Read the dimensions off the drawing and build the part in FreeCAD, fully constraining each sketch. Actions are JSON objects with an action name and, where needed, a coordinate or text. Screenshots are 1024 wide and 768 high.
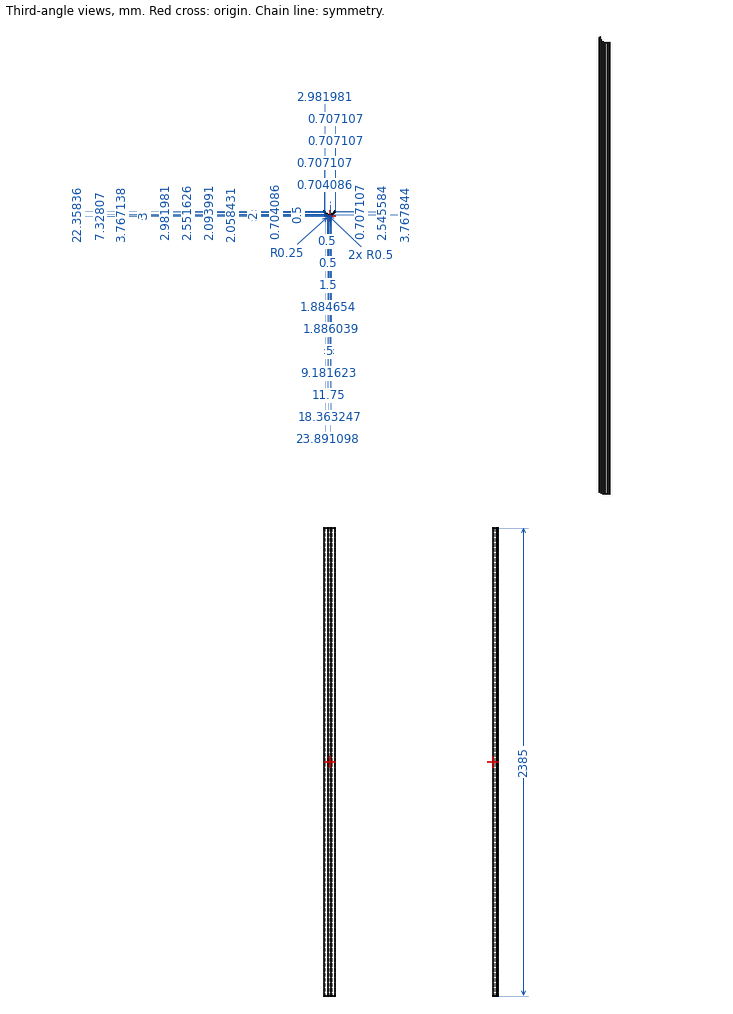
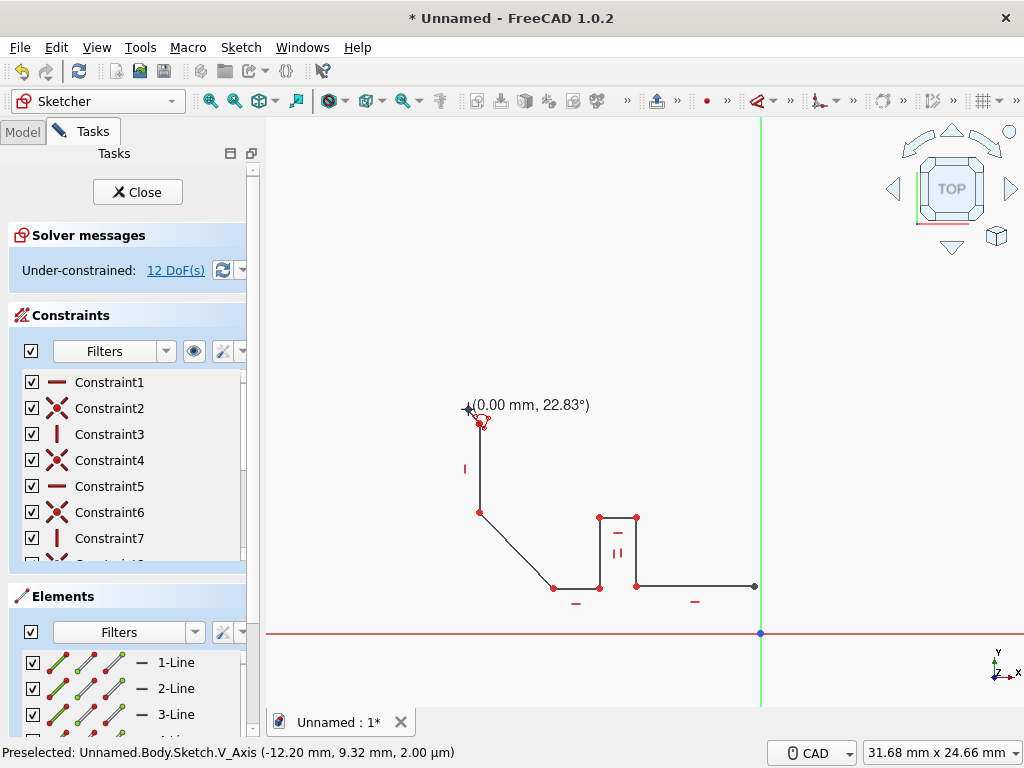
{"action": "scroll", "coordinate": [456, 409], "scroll_direction": "up", "scroll_amount": 2}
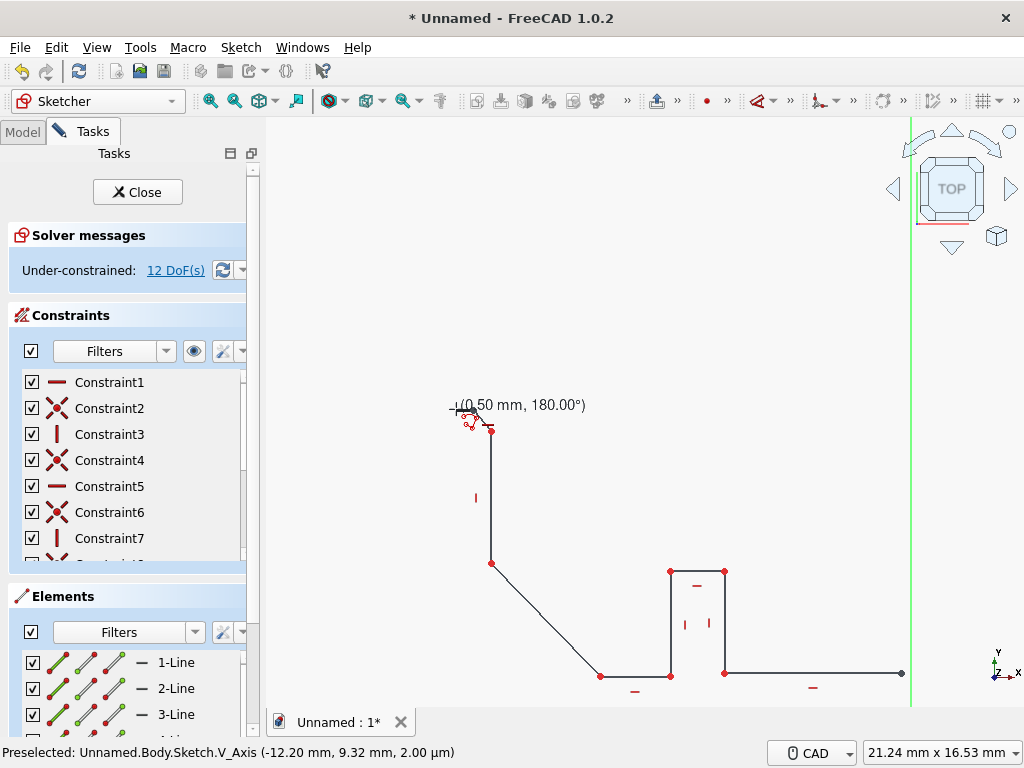
{"action": "left_click", "coordinate": [455, 409]}
{"action": "left_click", "coordinate": [455, 483]}
{"action": "right_click", "coordinate": [455, 483]}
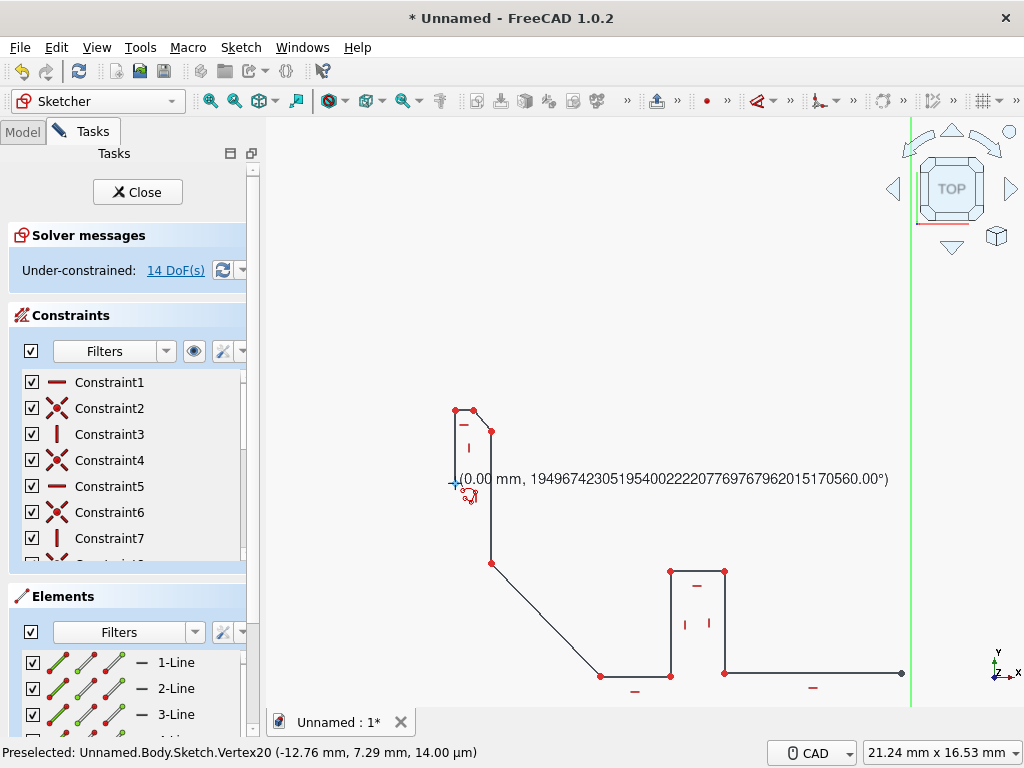
{"action": "left_click", "coordinate": [425, 495]}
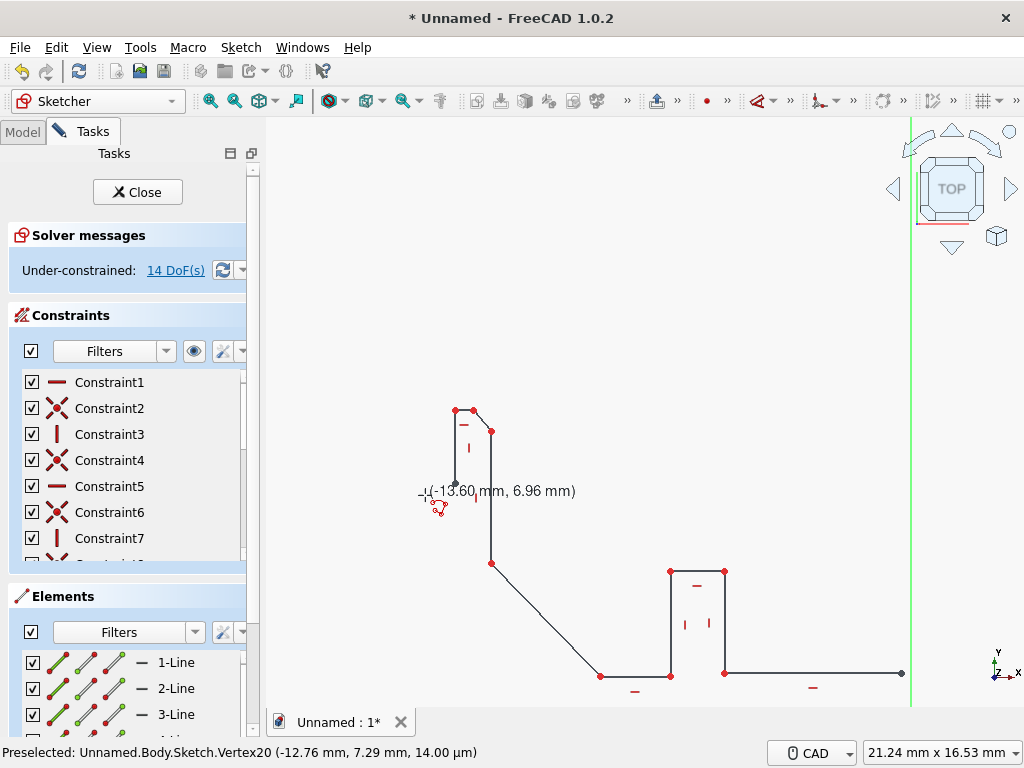
{"action": "scroll", "coordinate": [492, 429], "scroll_direction": "down", "scroll_amount": 8}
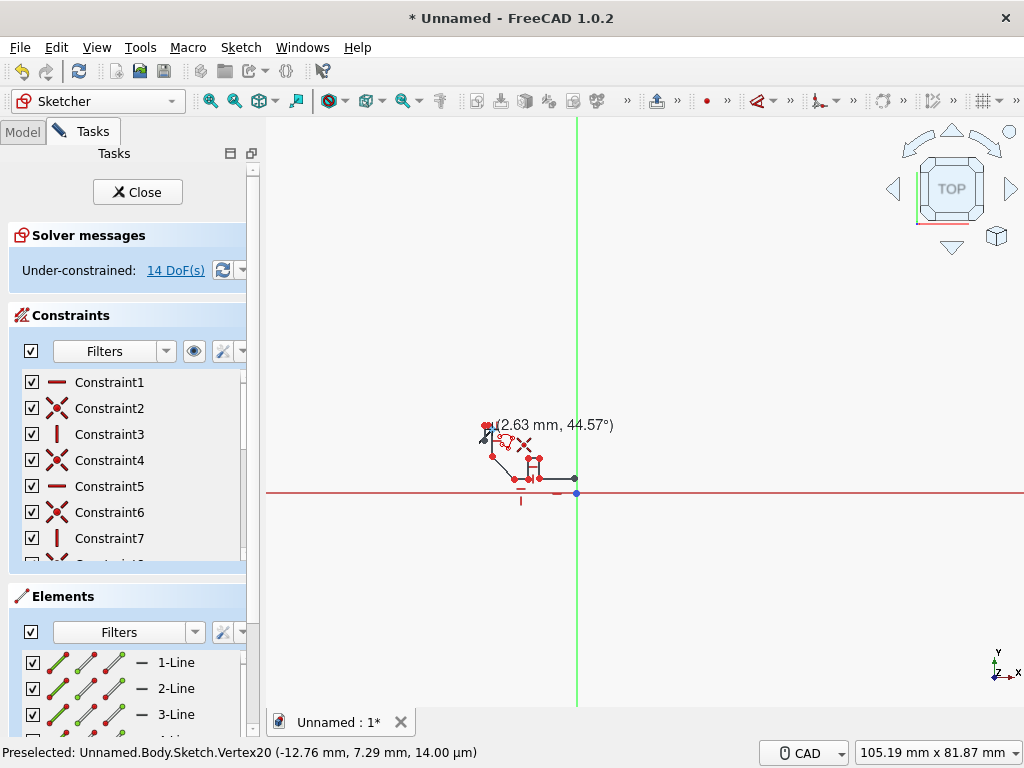
{"action": "left_click", "coordinate": [405, 369]}
{"action": "left_click", "coordinate": [405, 353]}
{"action": "left_click", "coordinate": [383, 332]}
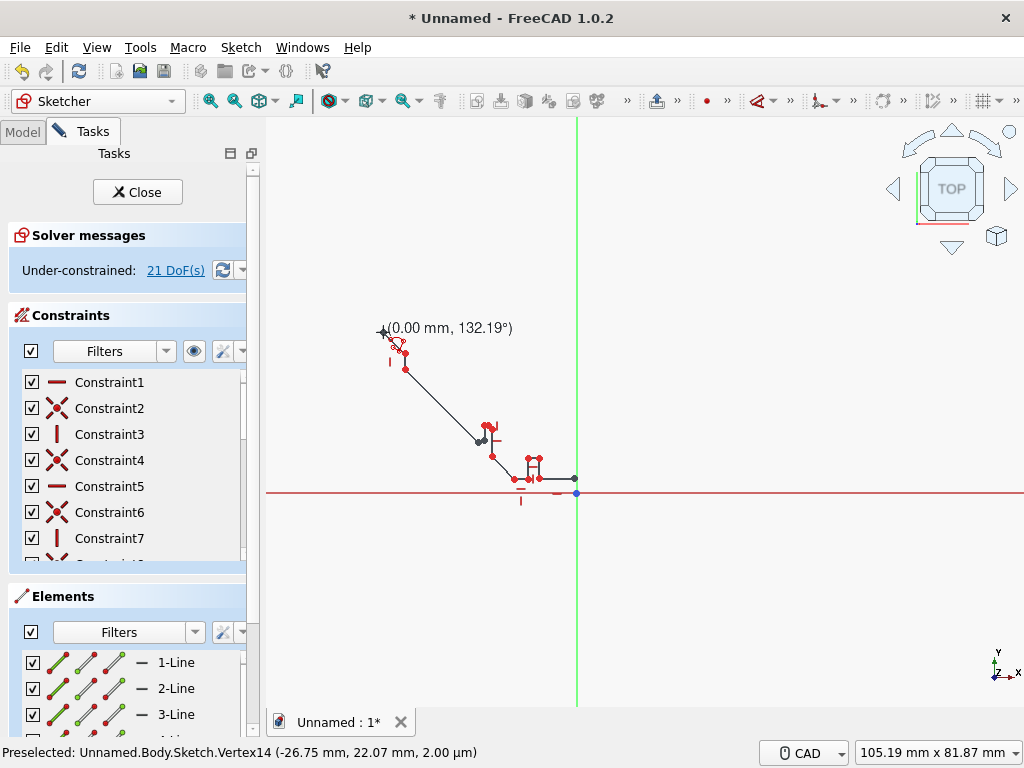
{"action": "scroll", "coordinate": [378, 332], "scroll_direction": "up", "scroll_amount": 6}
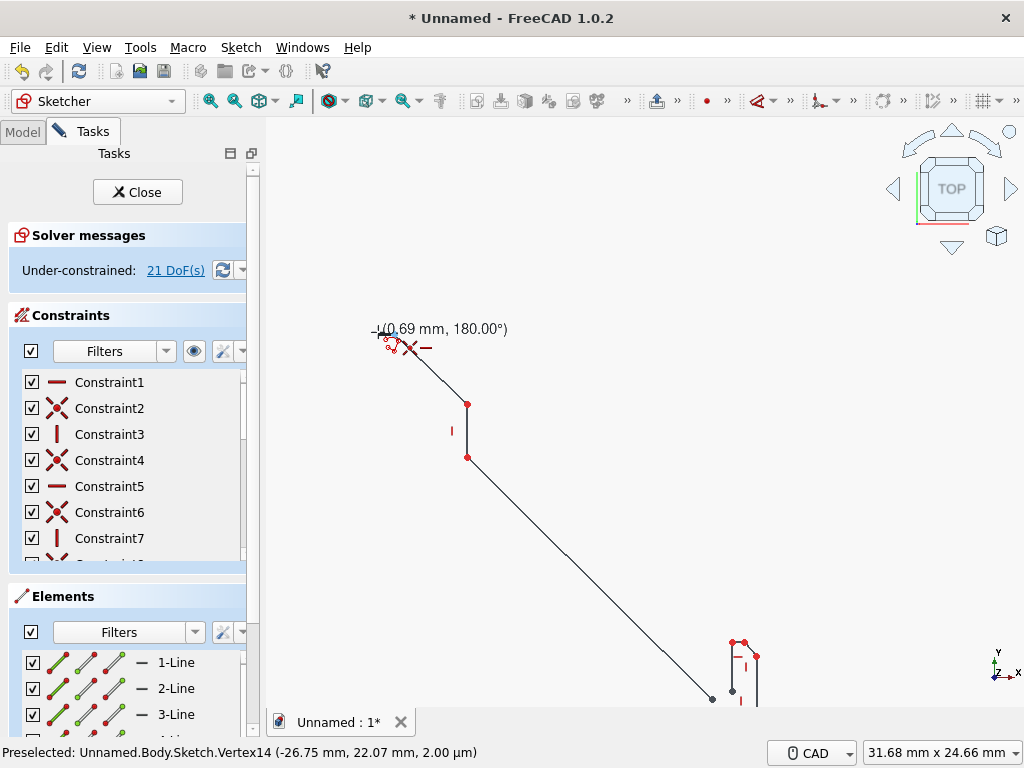
{"action": "left_click", "coordinate": [378, 331]}
{"action": "left_click", "coordinate": [361, 348]}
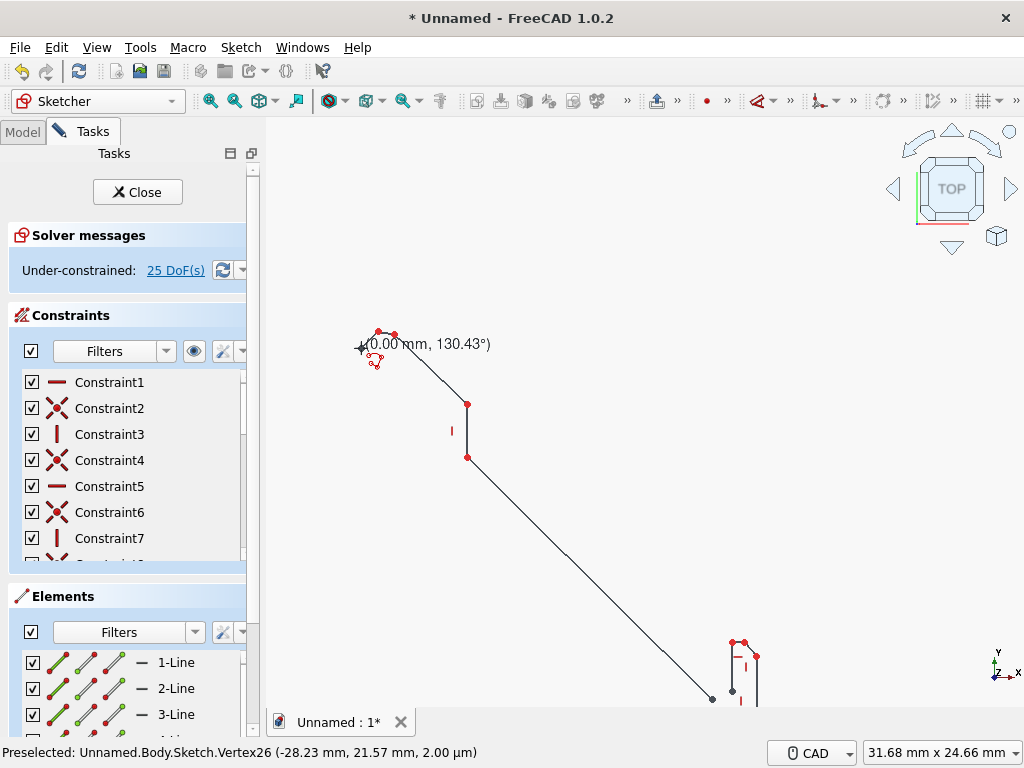
{"action": "scroll", "coordinate": [378, 332], "scroll_direction": "down", "scroll_amount": 6}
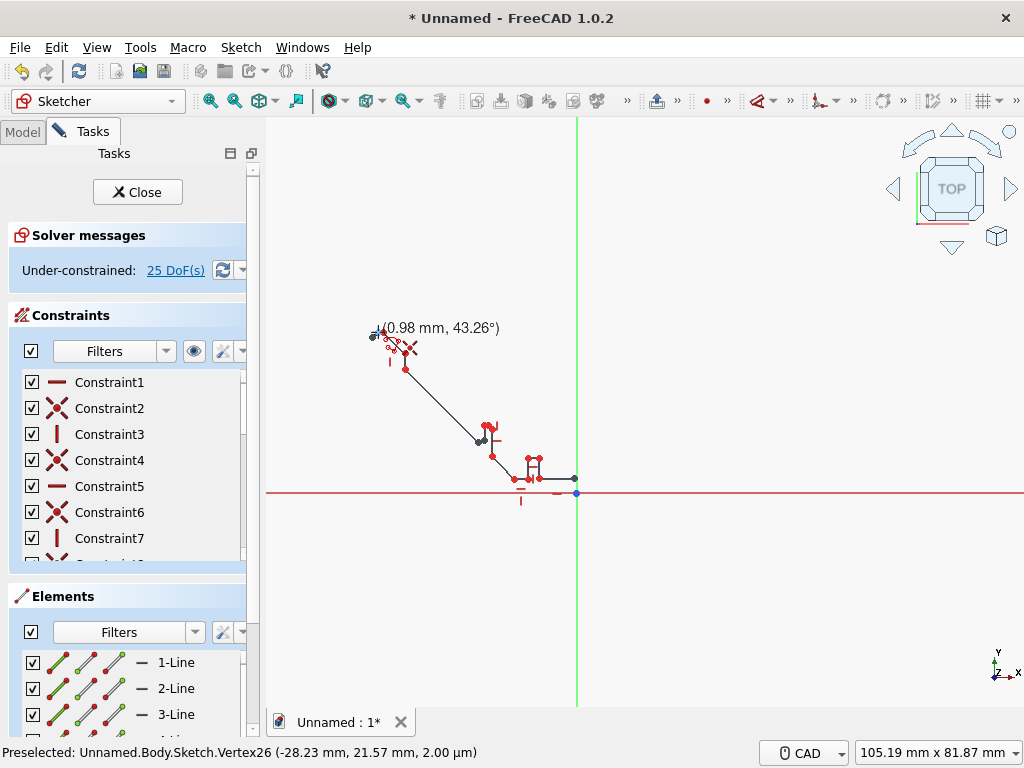
{"action": "left_click", "coordinate": [373, 355]}
{"action": "left_click", "coordinate": [511, 493]}
{"action": "left_click", "coordinate": [643, 484]}
{"action": "left_click", "coordinate": [781, 355]}
{"action": "left_click", "coordinate": [781, 337]}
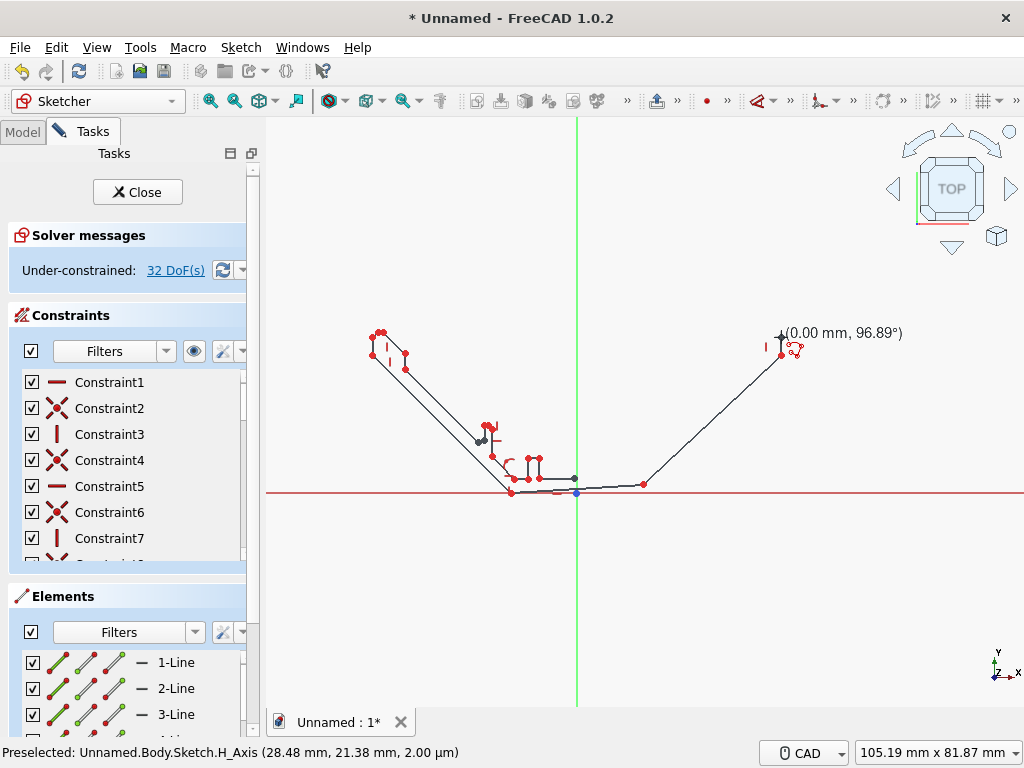
{"action": "scroll", "coordinate": [775, 332], "scroll_direction": "up", "scroll_amount": 4}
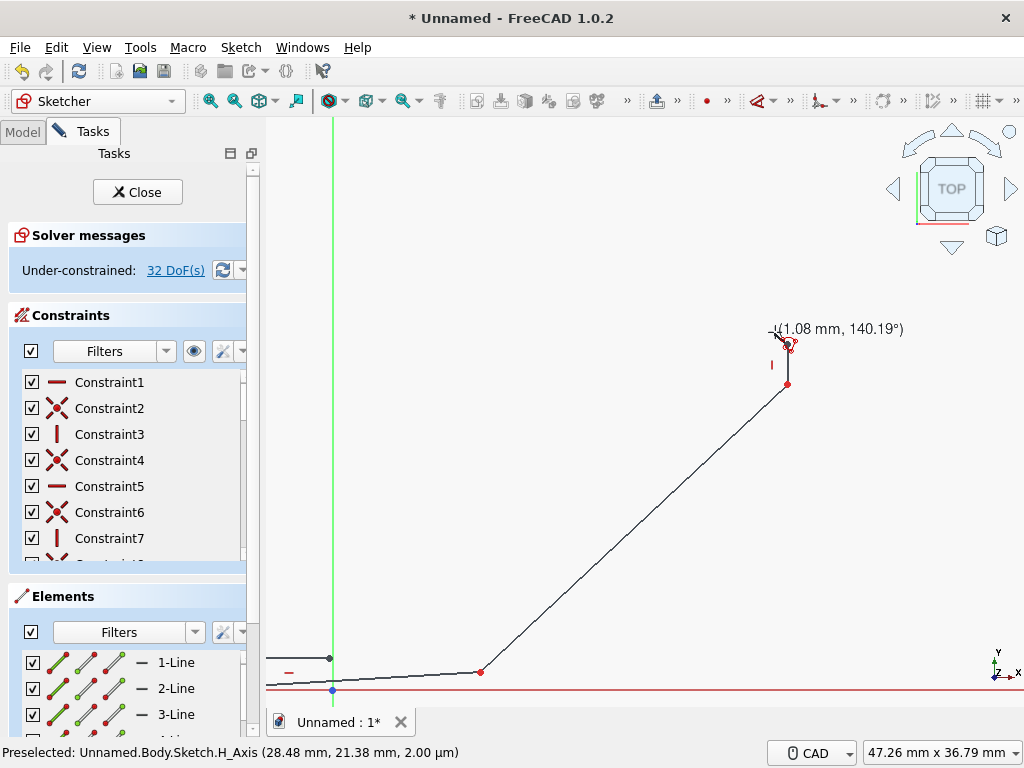
{"action": "left_click", "coordinate": [775, 331]}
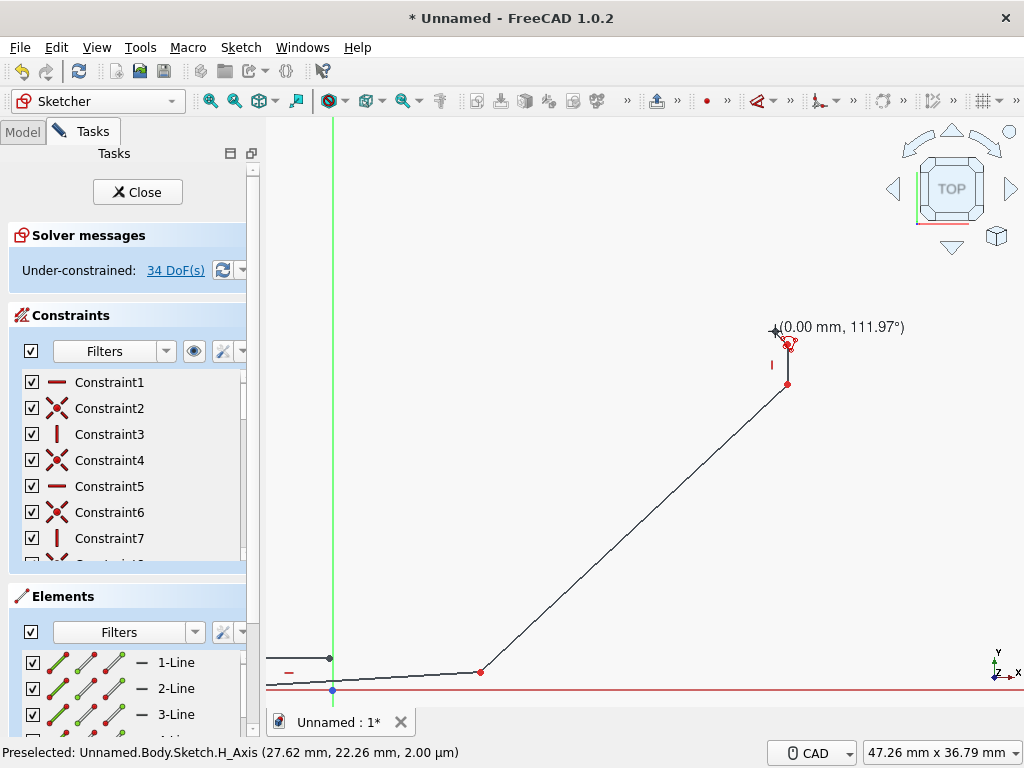
{"action": "scroll", "coordinate": [764, 331], "scroll_direction": "up", "scroll_amount": 2}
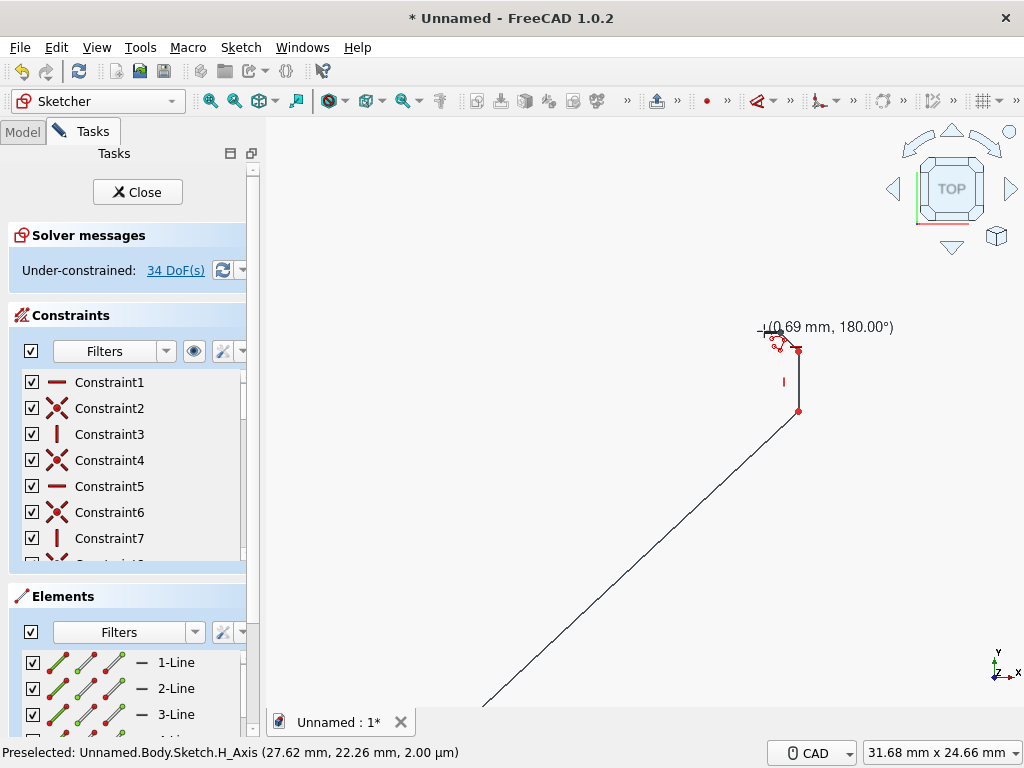
{"action": "left_click", "coordinate": [764, 331]}